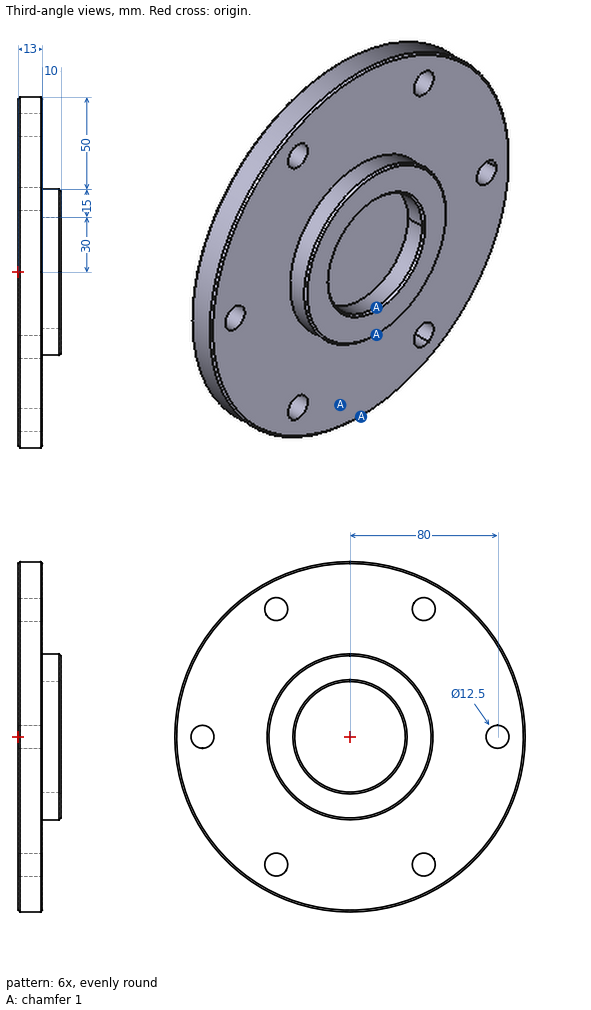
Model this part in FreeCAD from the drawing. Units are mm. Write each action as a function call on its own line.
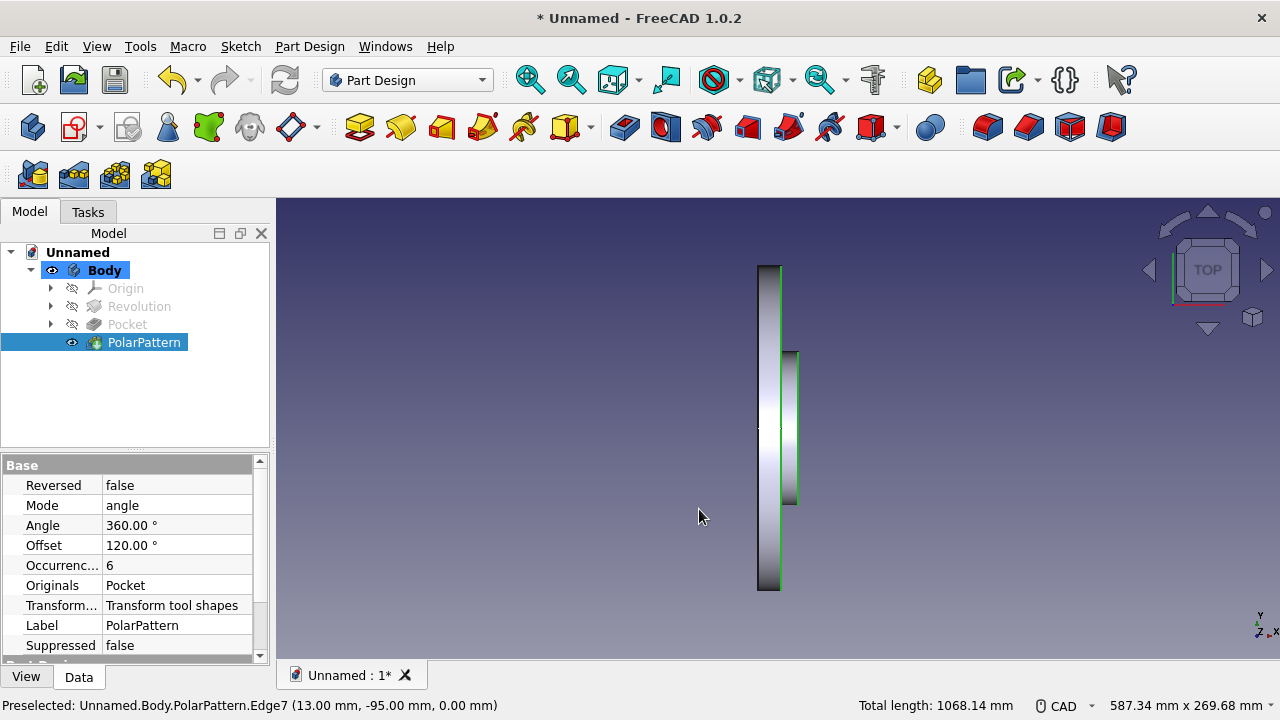
click(758, 559, ctrl)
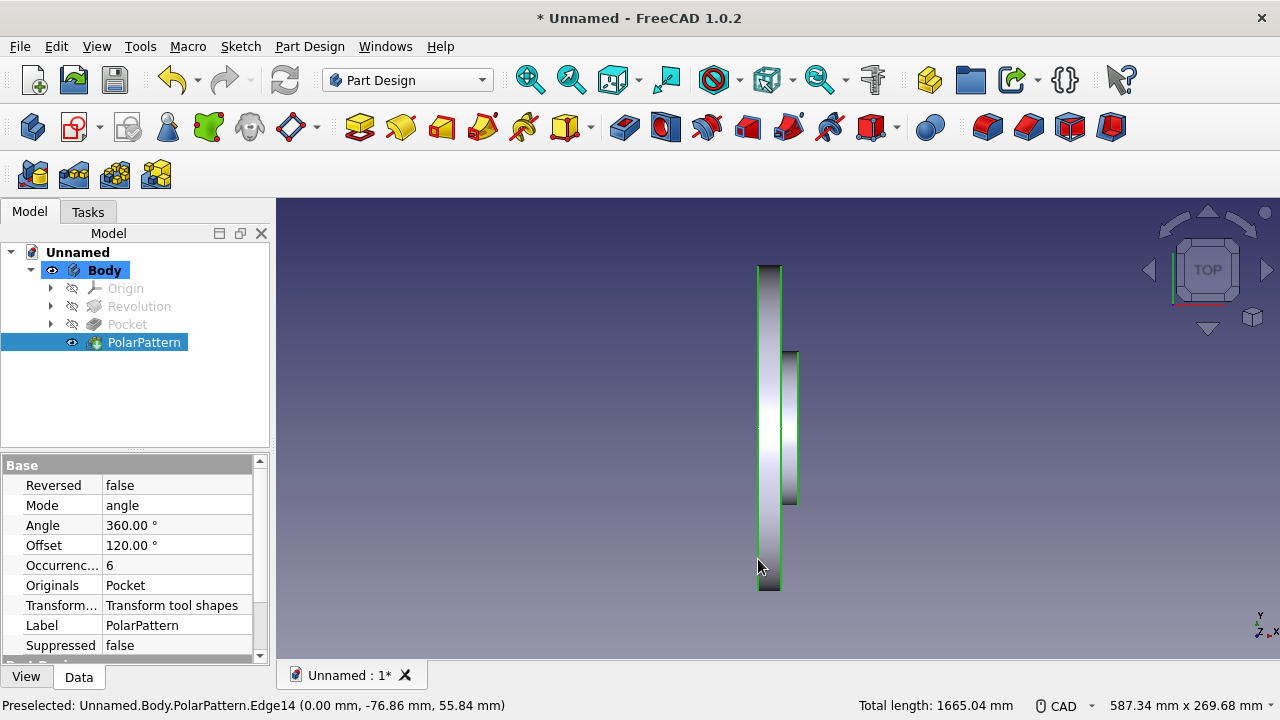
click(1029, 128)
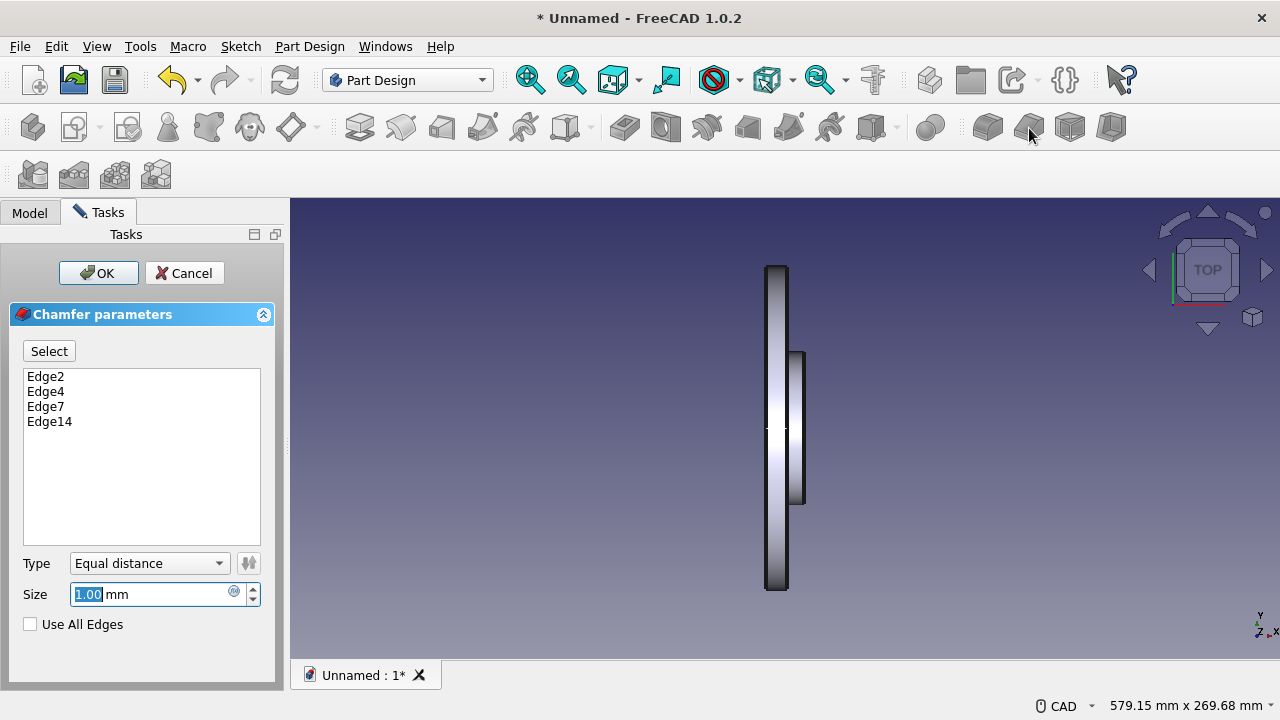
text(1)
key(Tab)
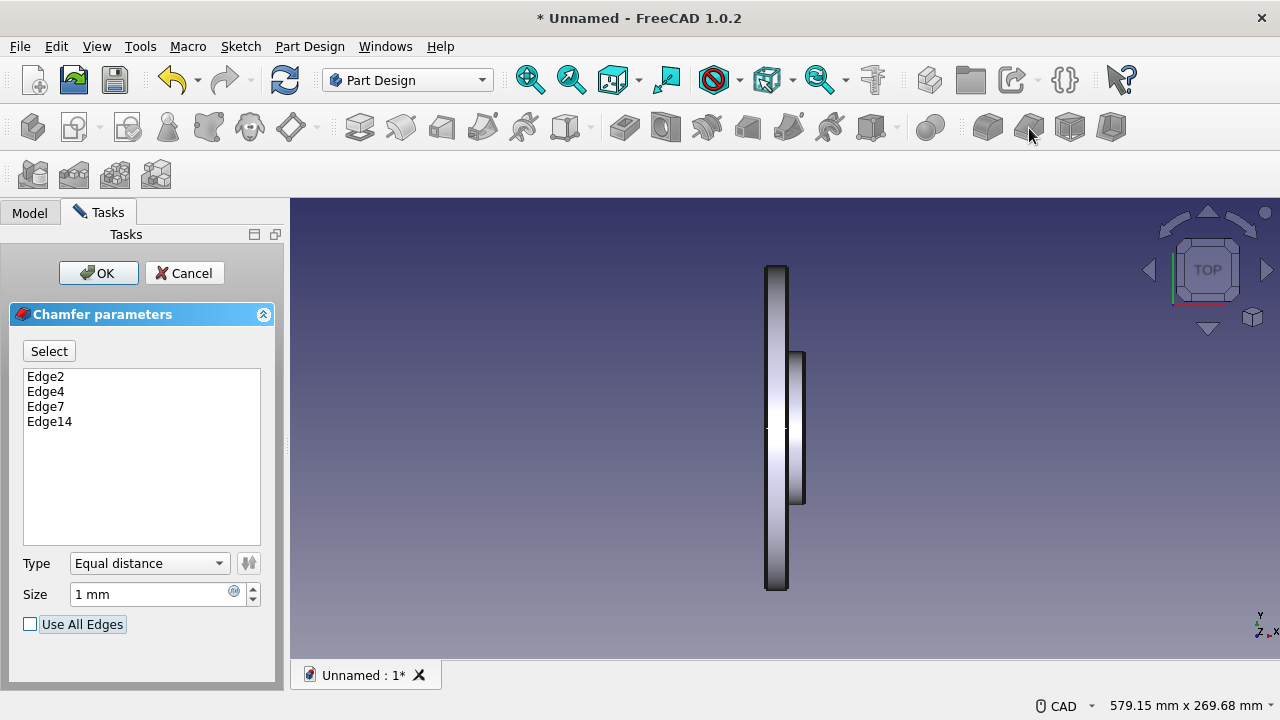
click(99, 273)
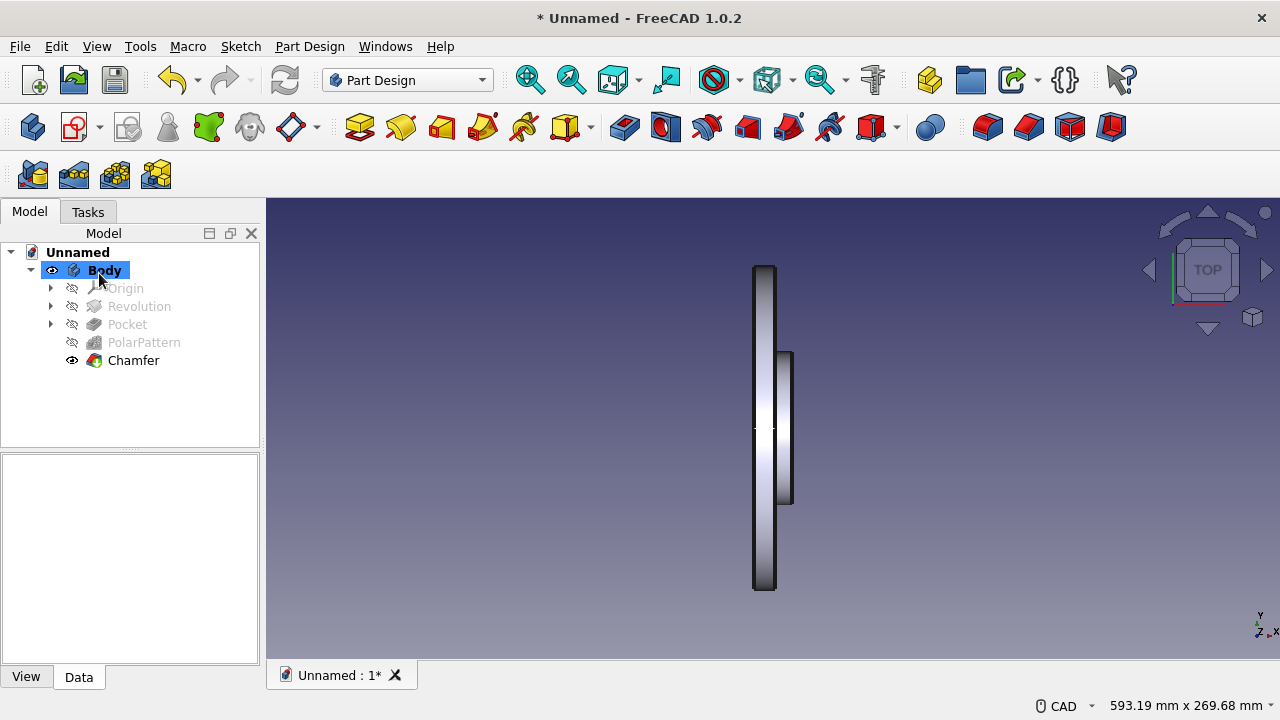
key(0)